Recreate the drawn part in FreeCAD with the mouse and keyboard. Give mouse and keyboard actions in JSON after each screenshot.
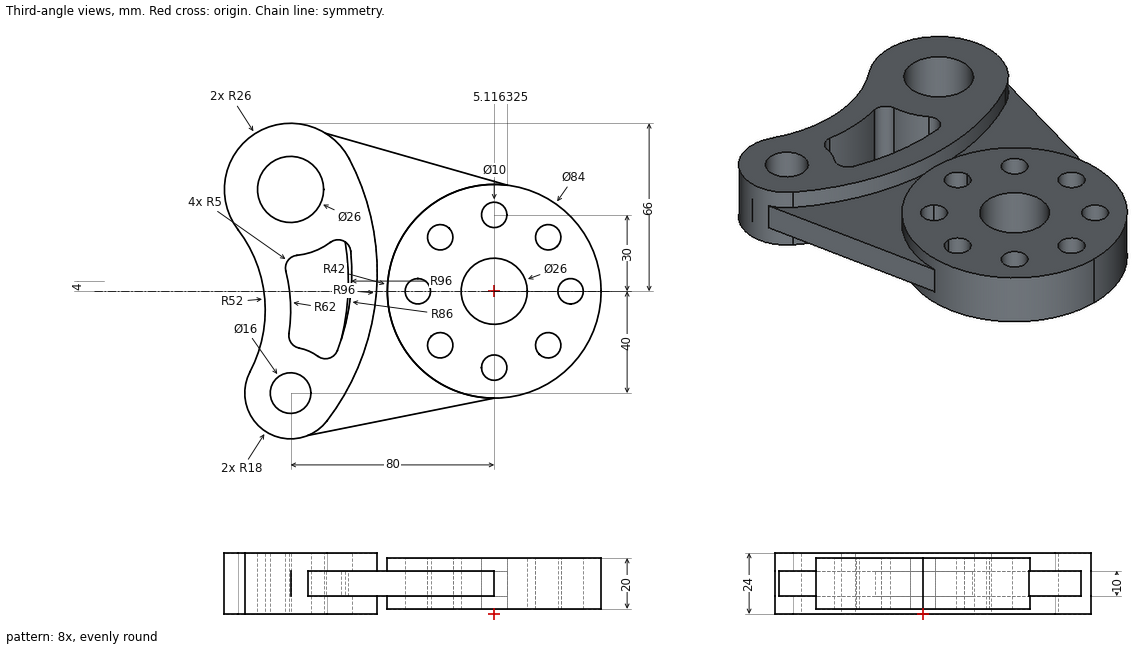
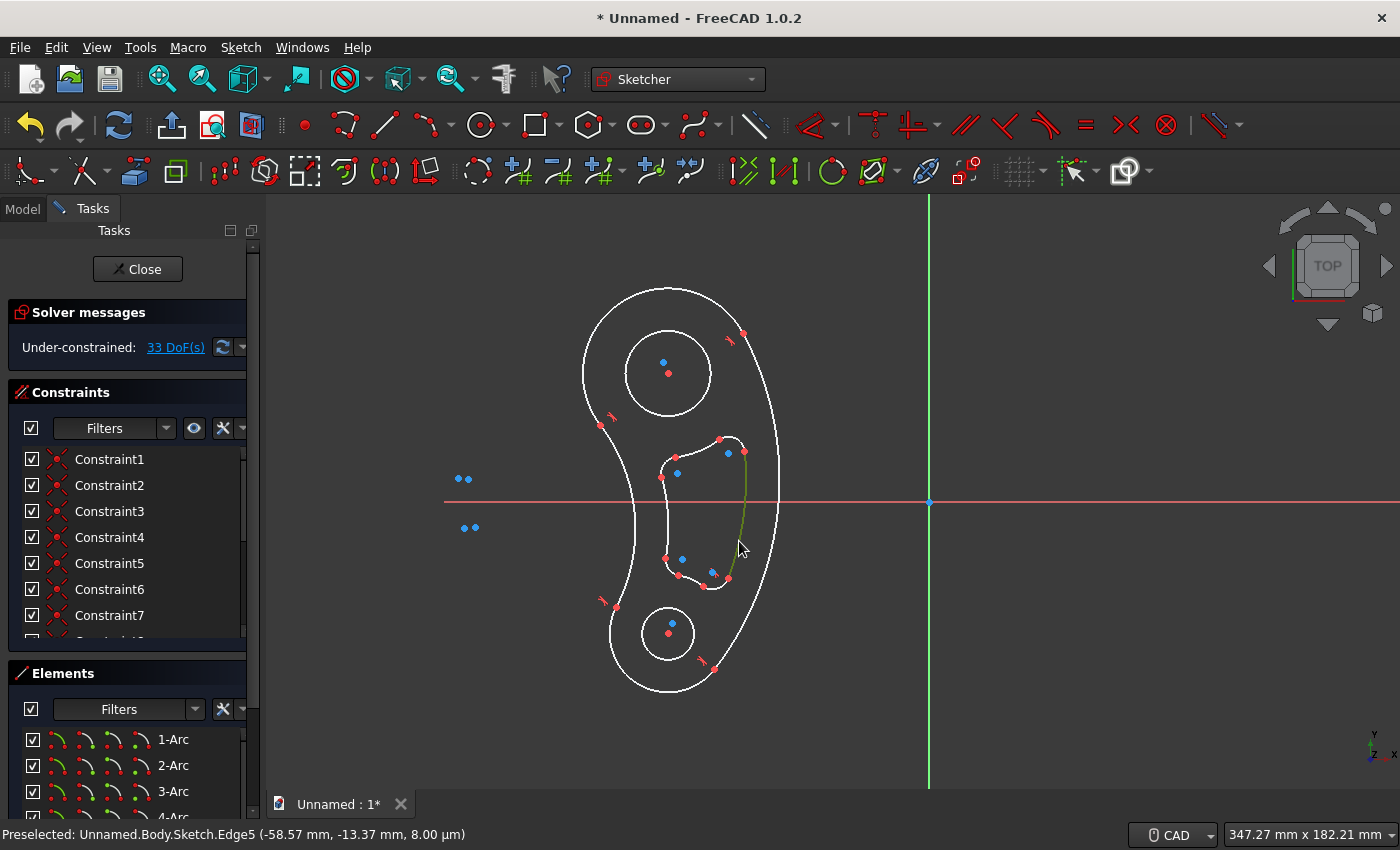
{"action": "scroll", "coordinate": [741, 442], "scroll_direction": "up", "scroll_amount": 2}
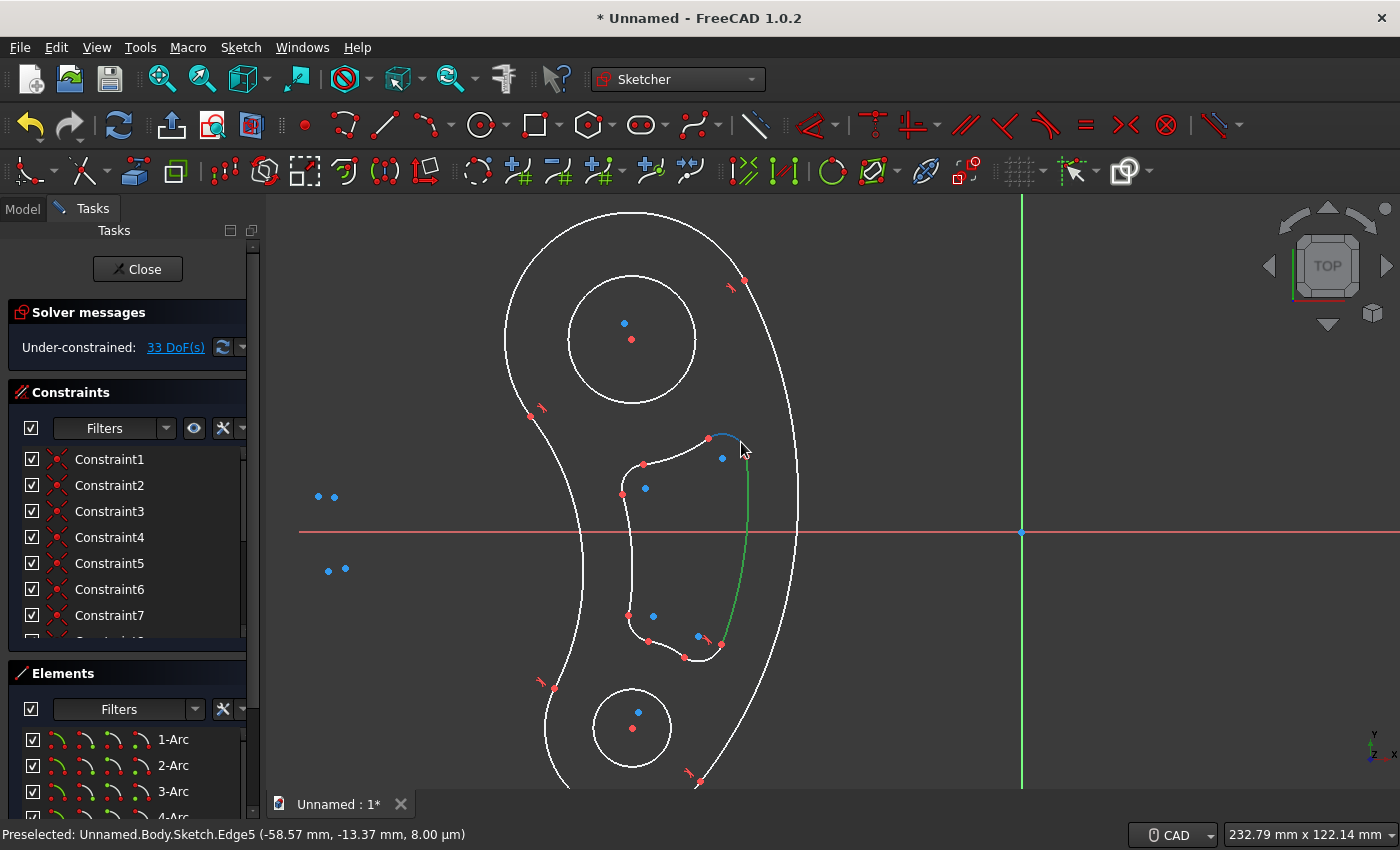
{"action": "left_click", "coordinate": [741, 442]}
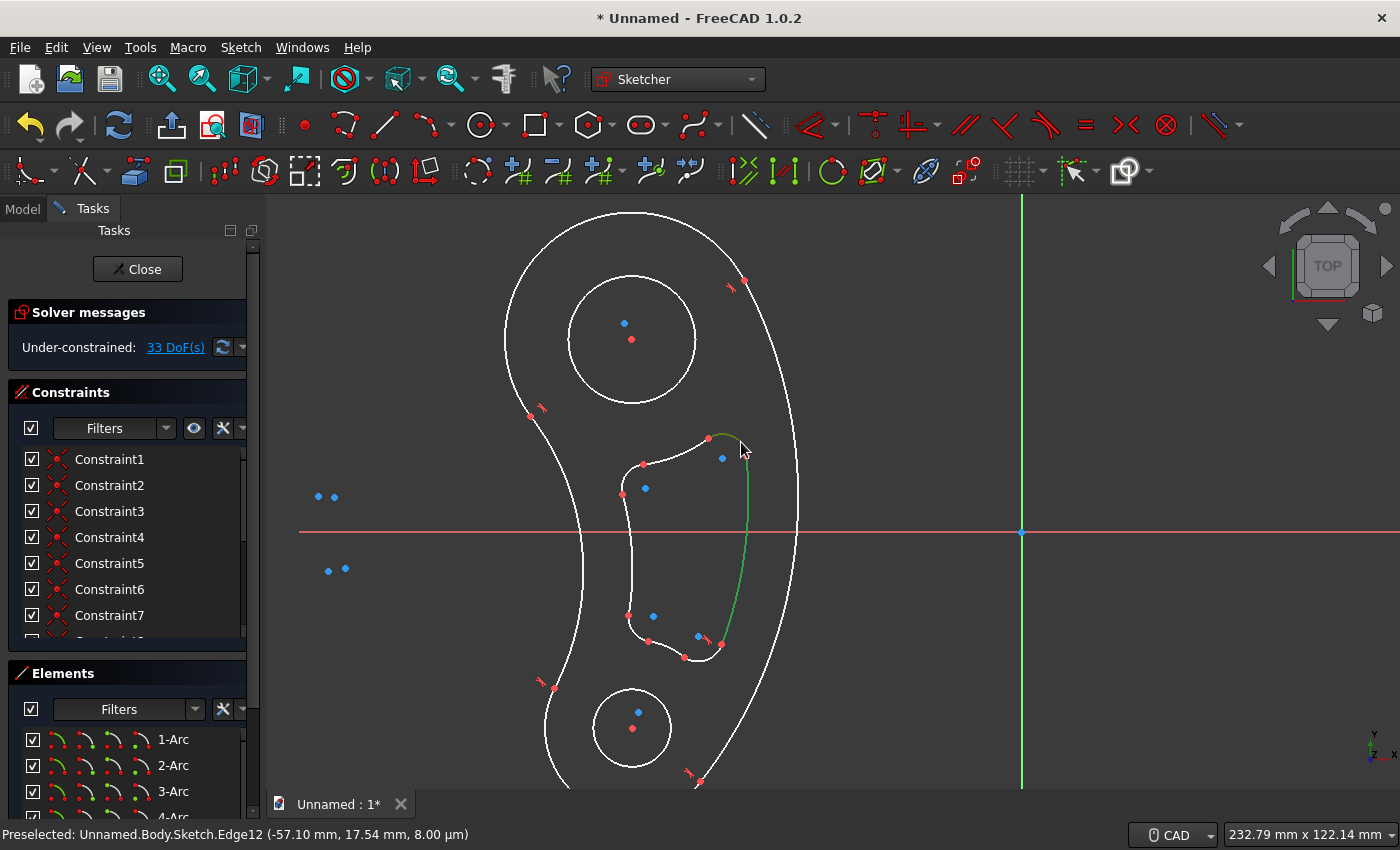
{"action": "left_click", "coordinate": [1046, 126]}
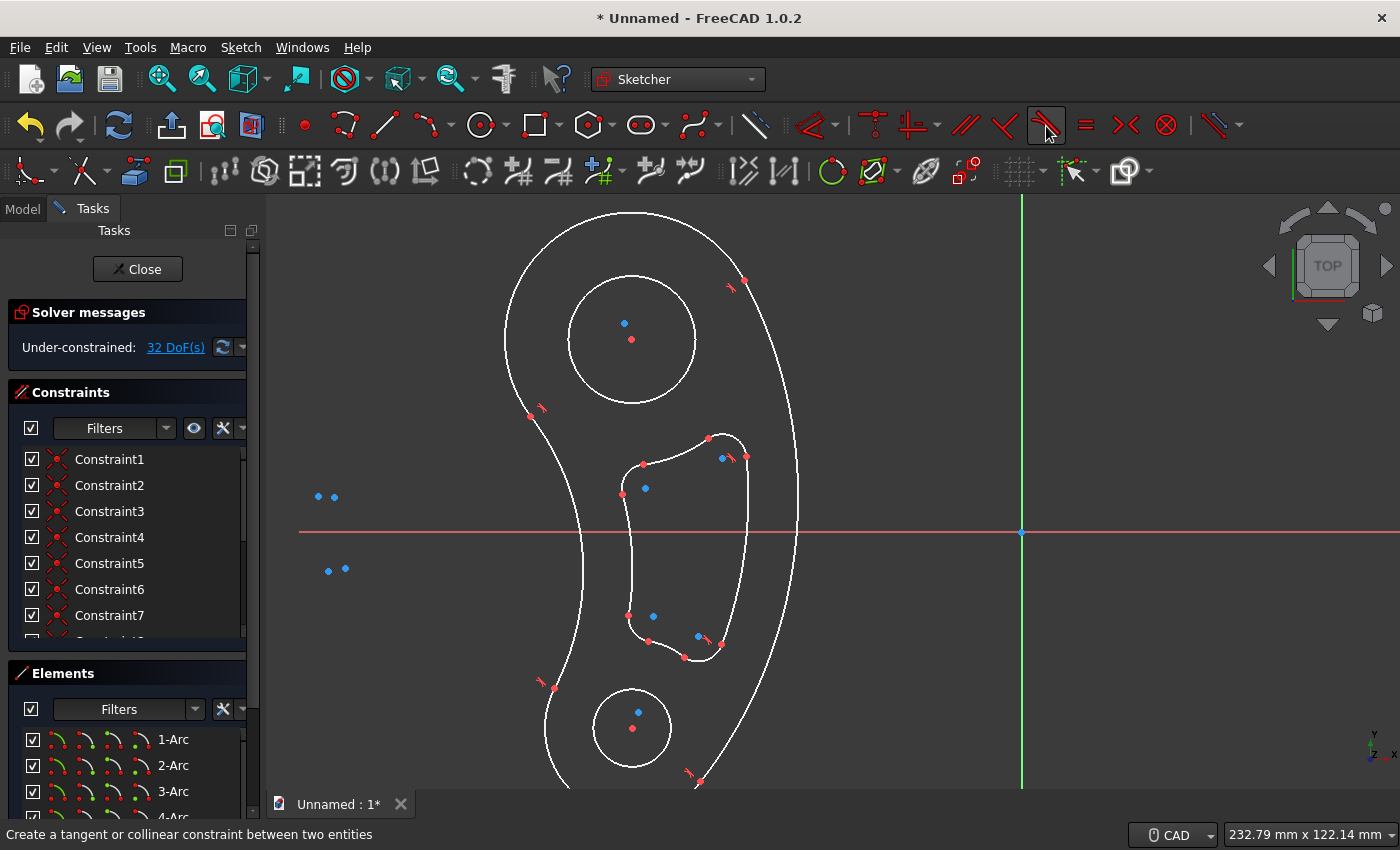
{"action": "left_click", "coordinate": [697, 661]}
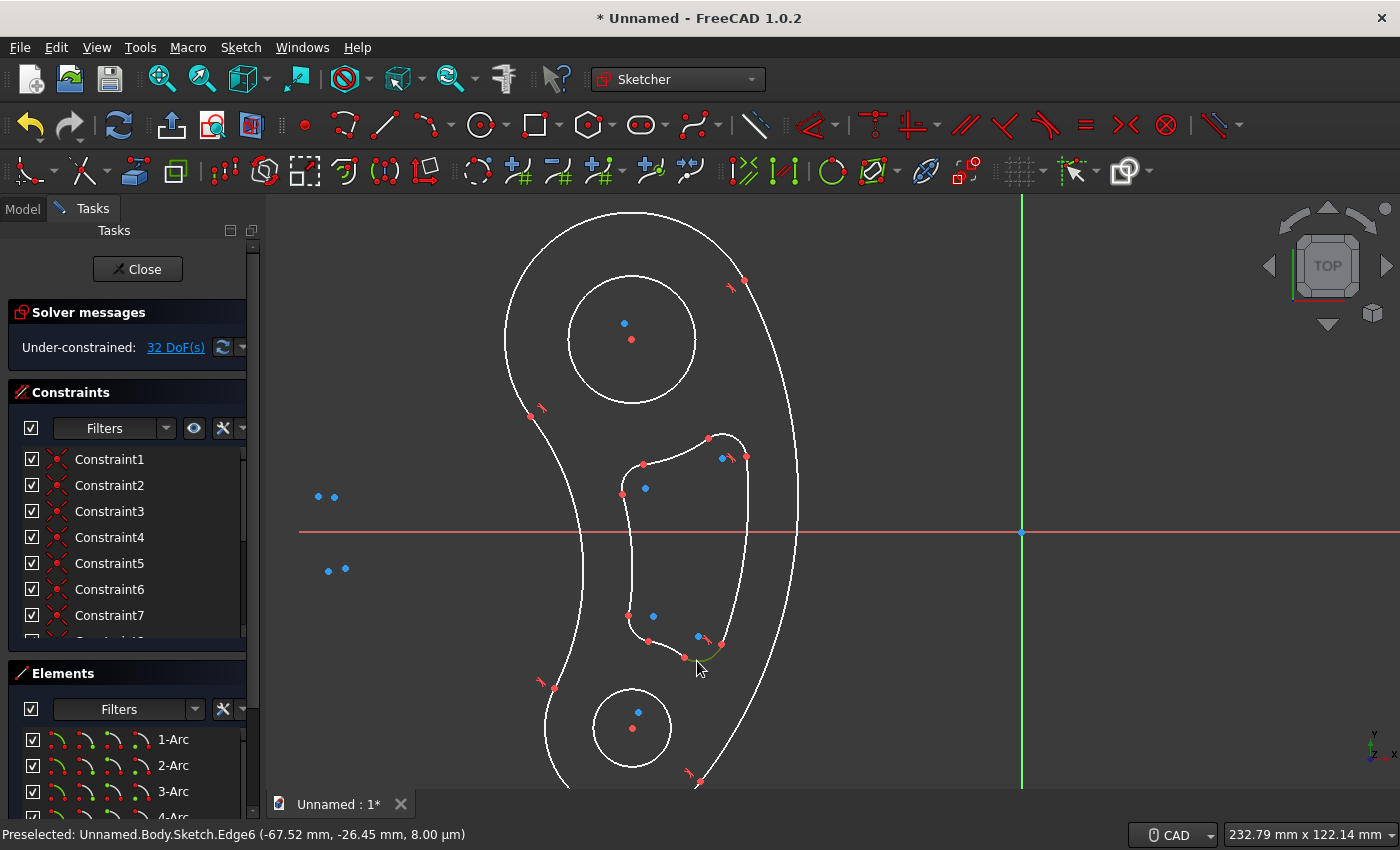
{"action": "left_click", "coordinate": [675, 650]}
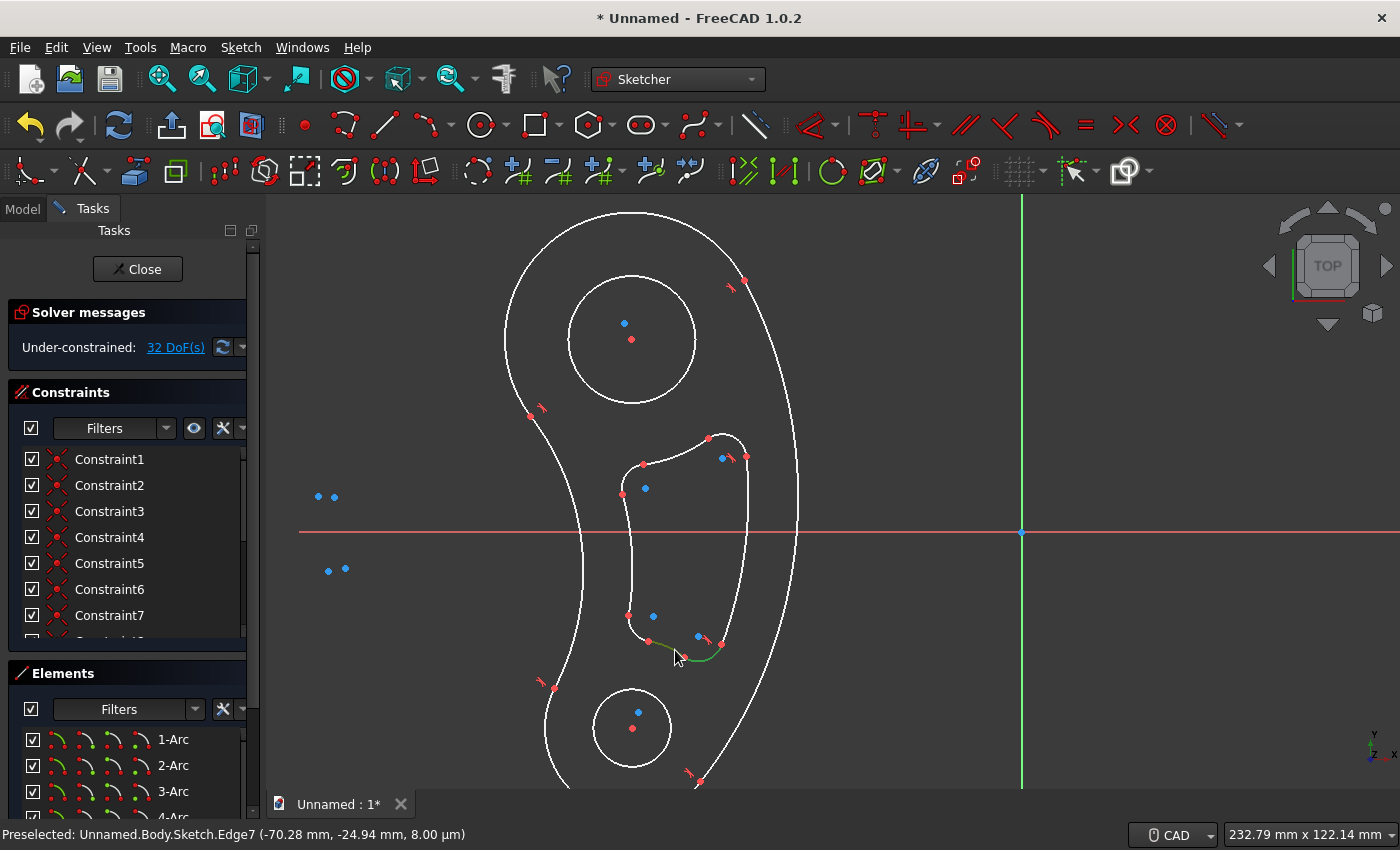
{"action": "left_click", "coordinate": [1046, 126]}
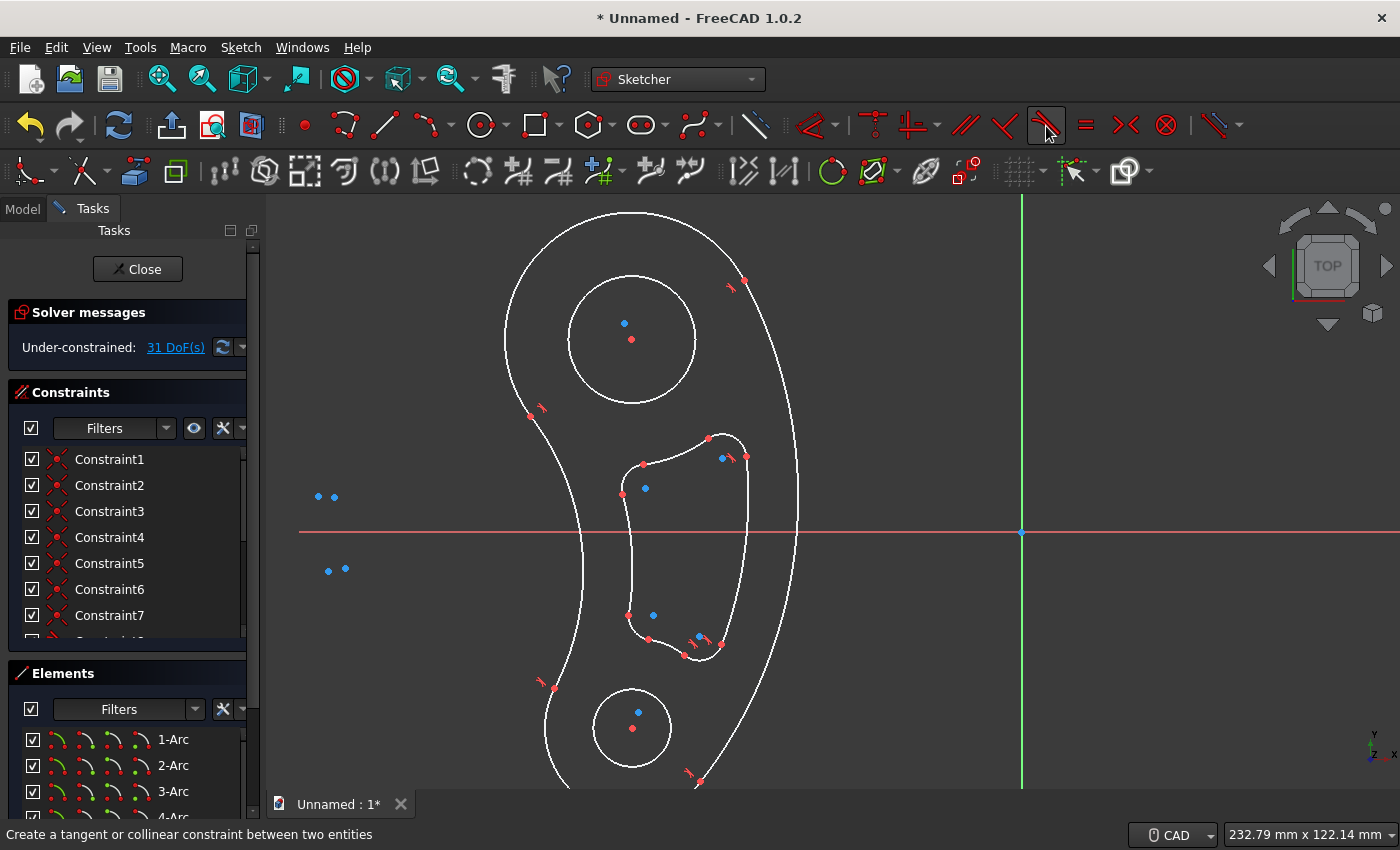
{"action": "left_click", "coordinate": [674, 649]}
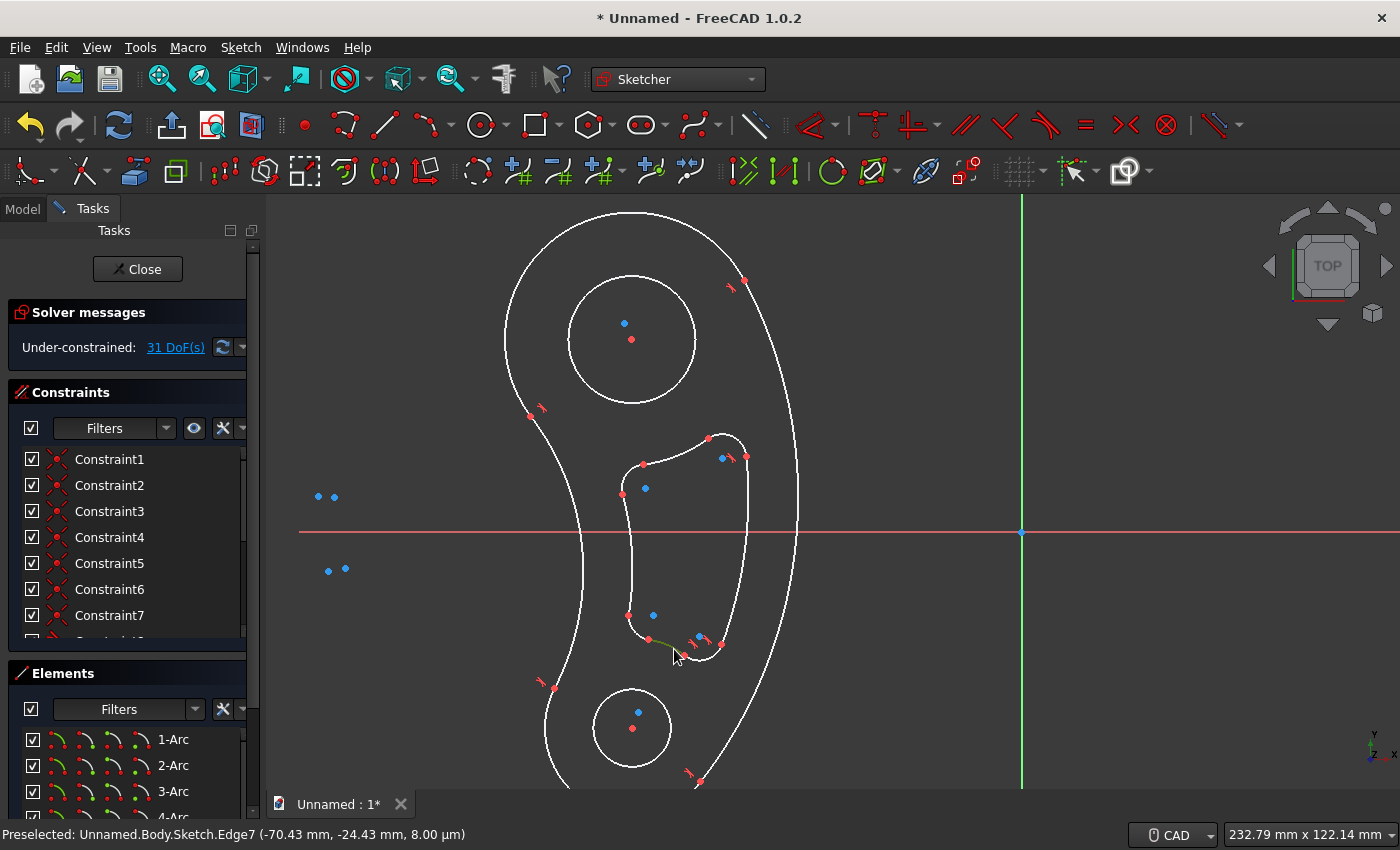
{"action": "scroll", "coordinate": [631, 625], "scroll_direction": "up", "scroll_amount": 2}